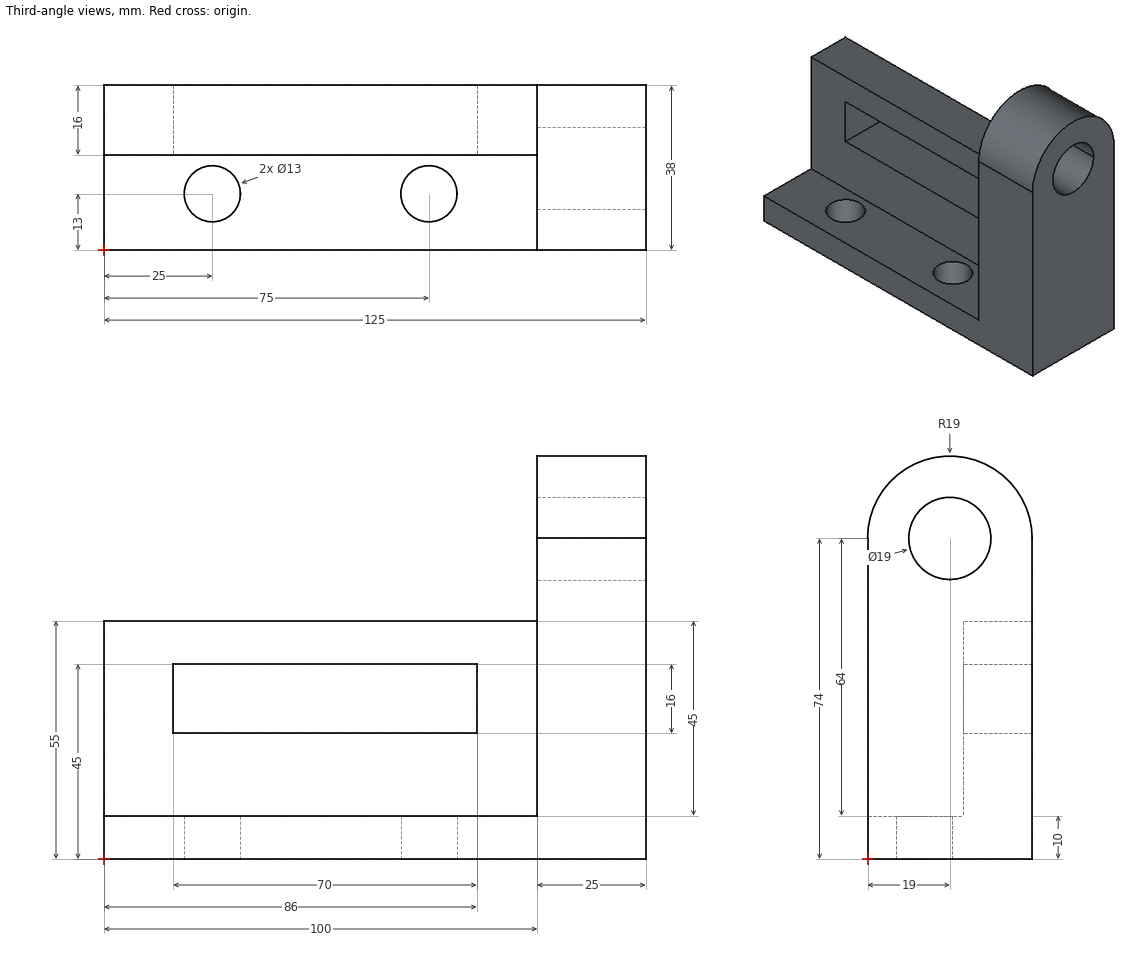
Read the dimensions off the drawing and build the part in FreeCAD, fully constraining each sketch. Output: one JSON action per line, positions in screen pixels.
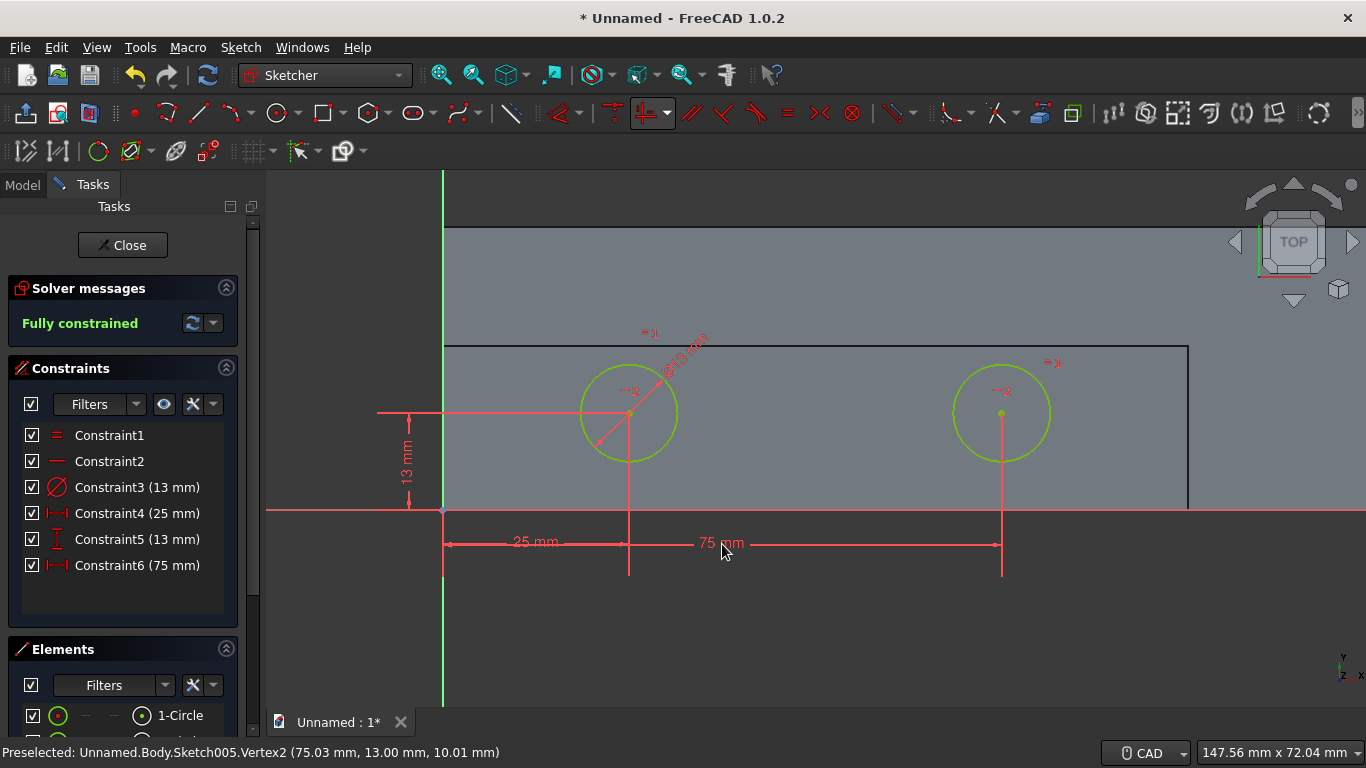
{"action": "left_click", "coordinate": [123, 245]}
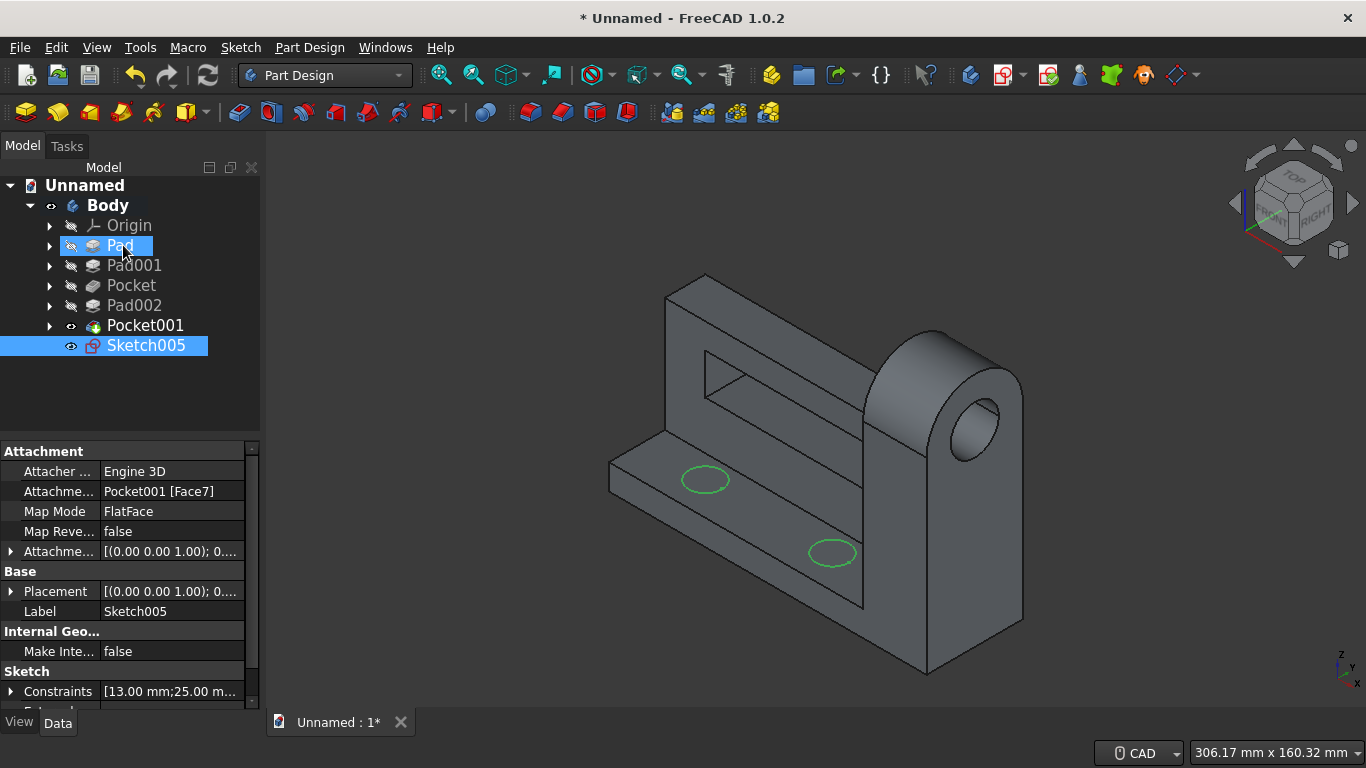
{"action": "left_click", "coordinate": [240, 112]}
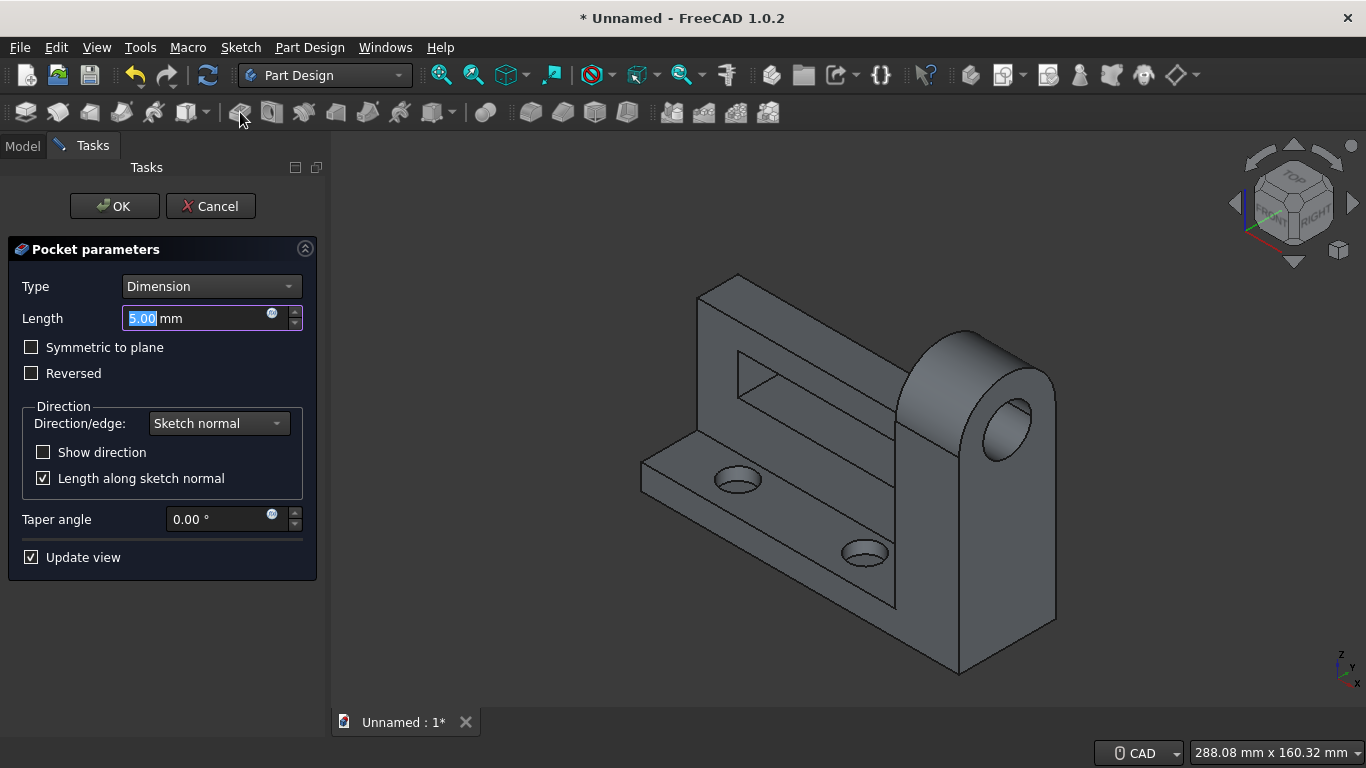
{"action": "type", "text": "10"}
{"action": "key", "text": "Tab"}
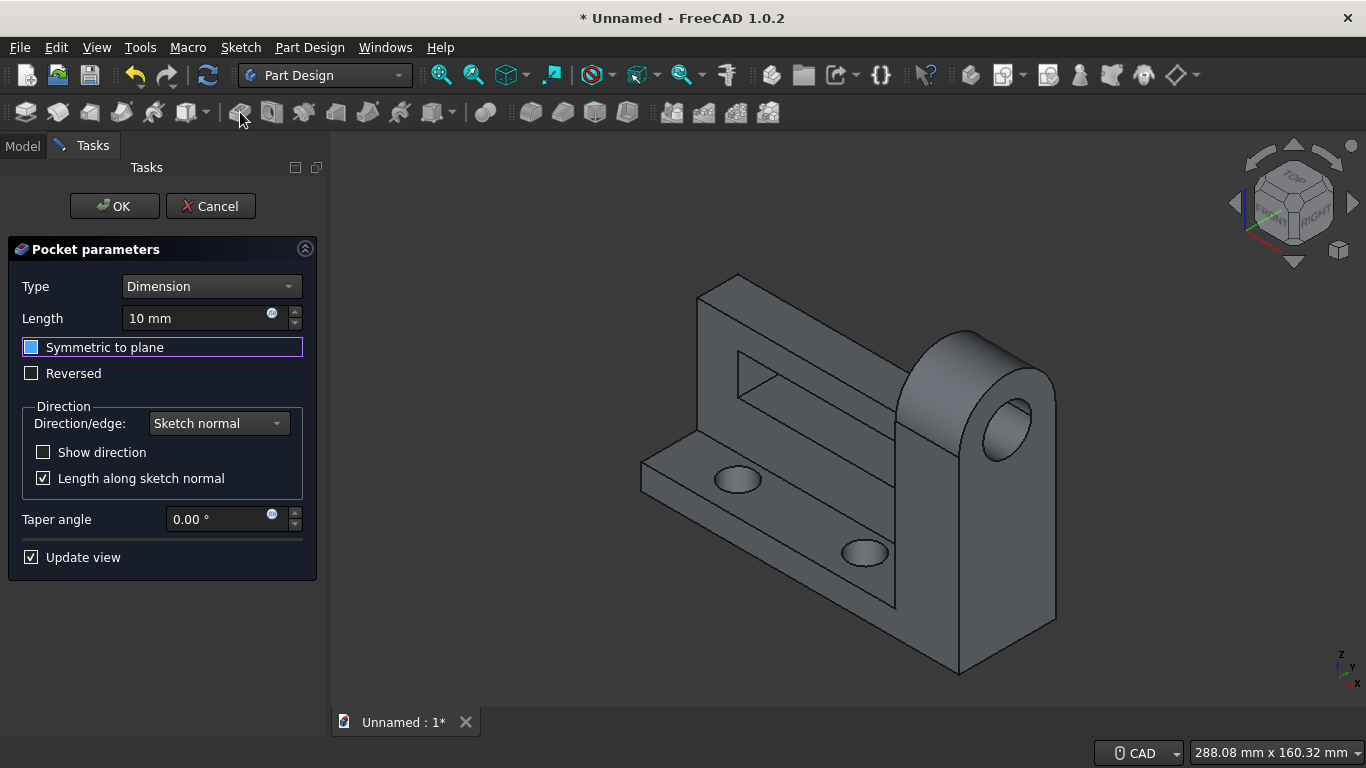
{"action": "left_click", "coordinate": [115, 206]}